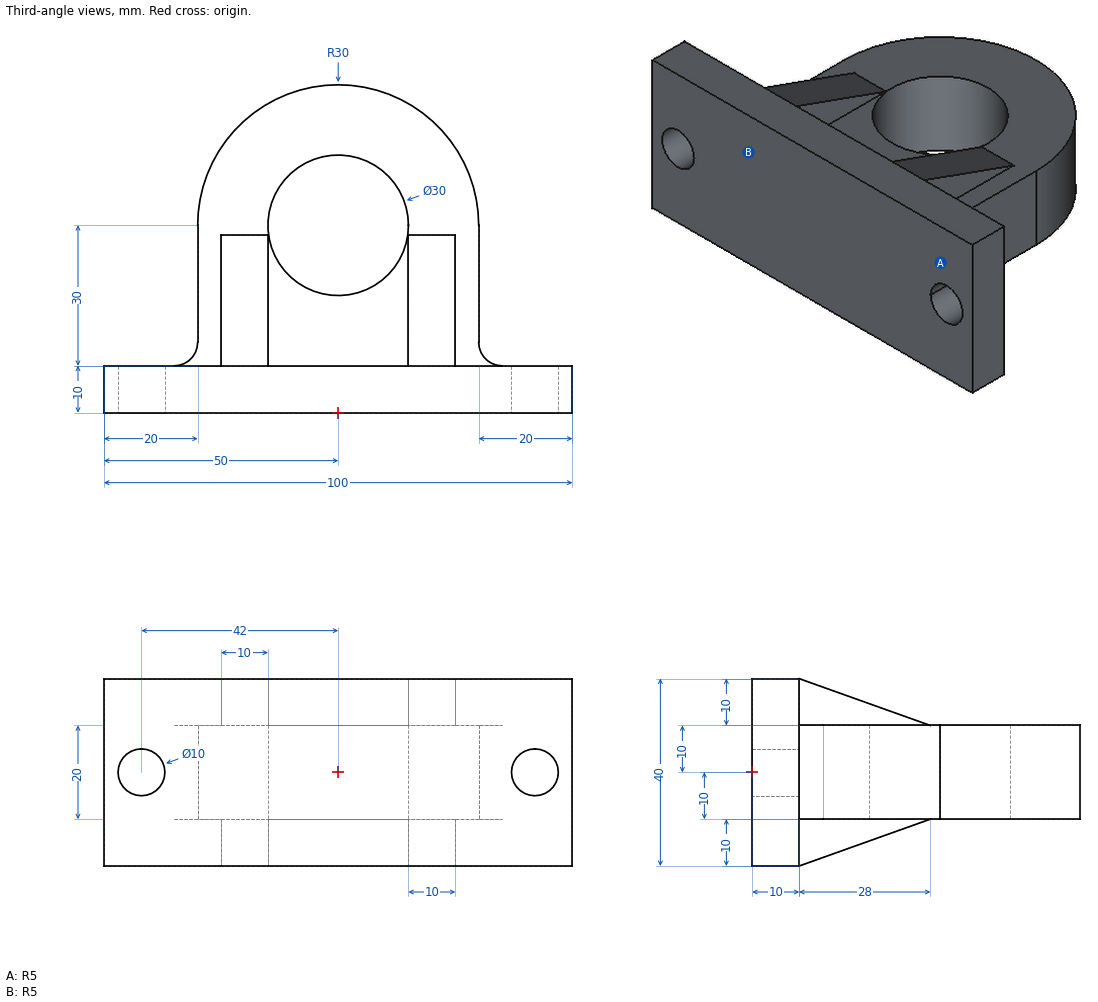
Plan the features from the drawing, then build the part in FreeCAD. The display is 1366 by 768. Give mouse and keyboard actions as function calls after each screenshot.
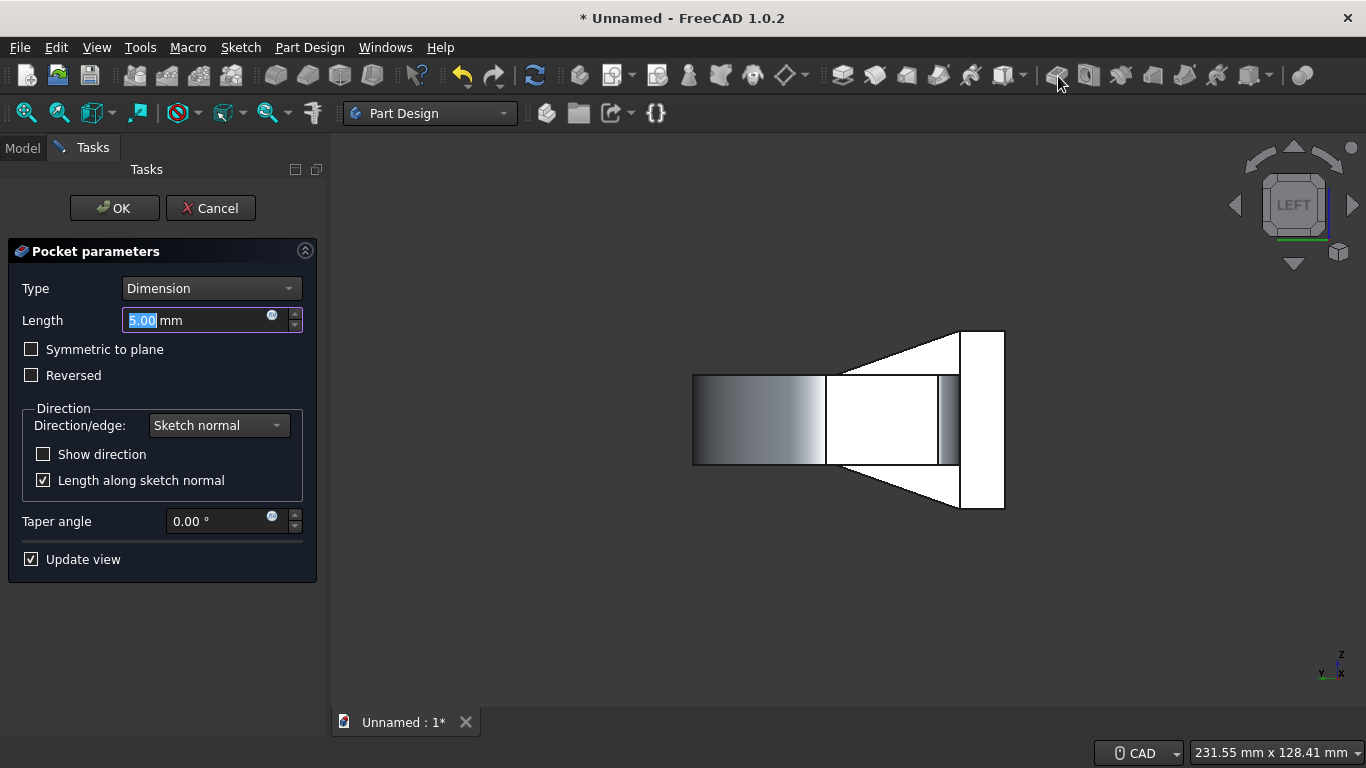
click(212, 288)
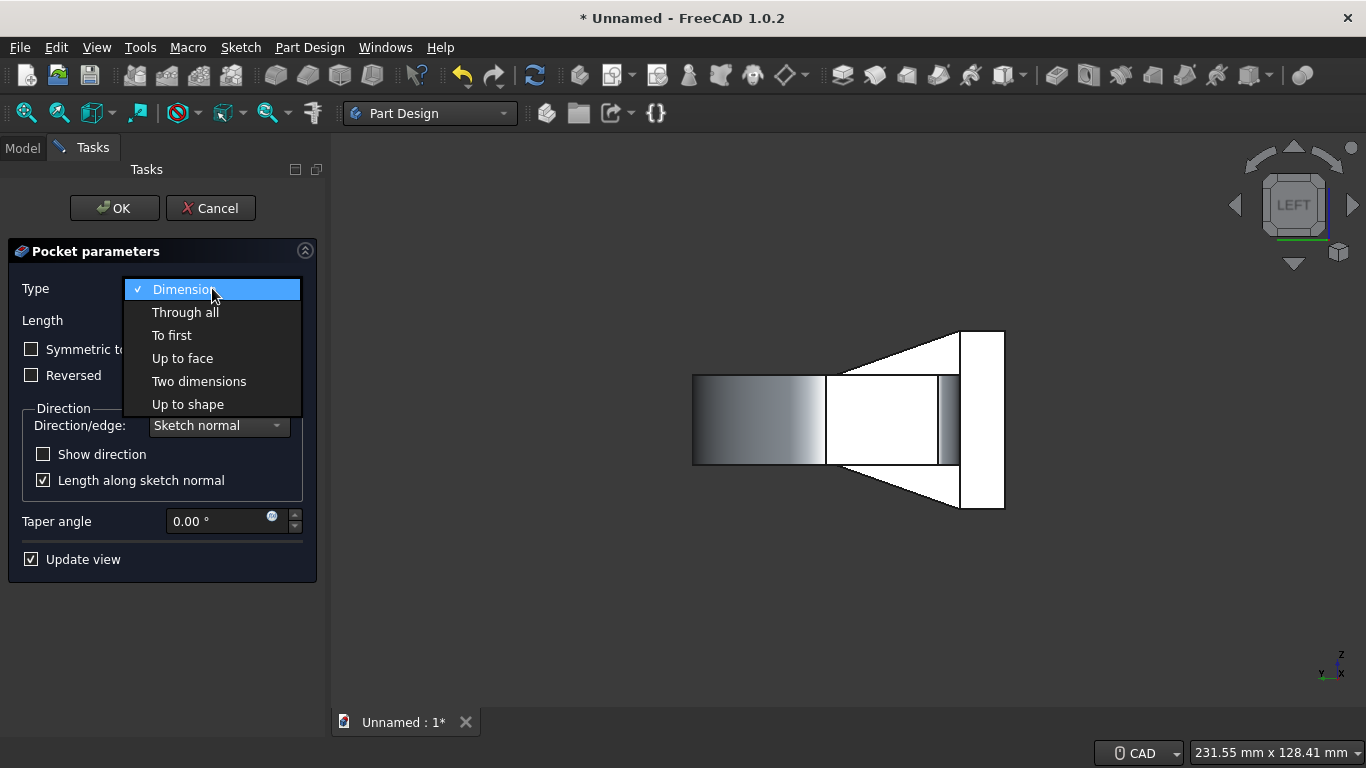
click(212, 312)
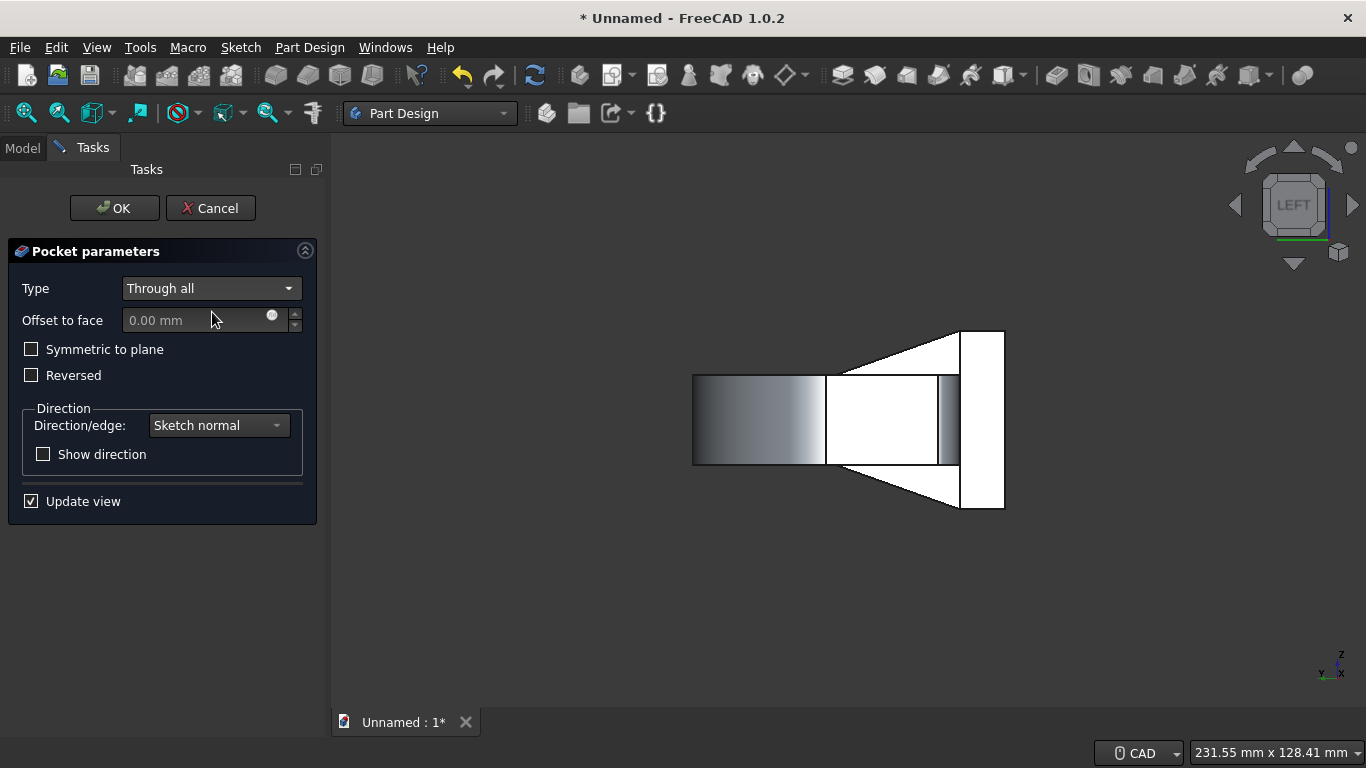
click(115, 208)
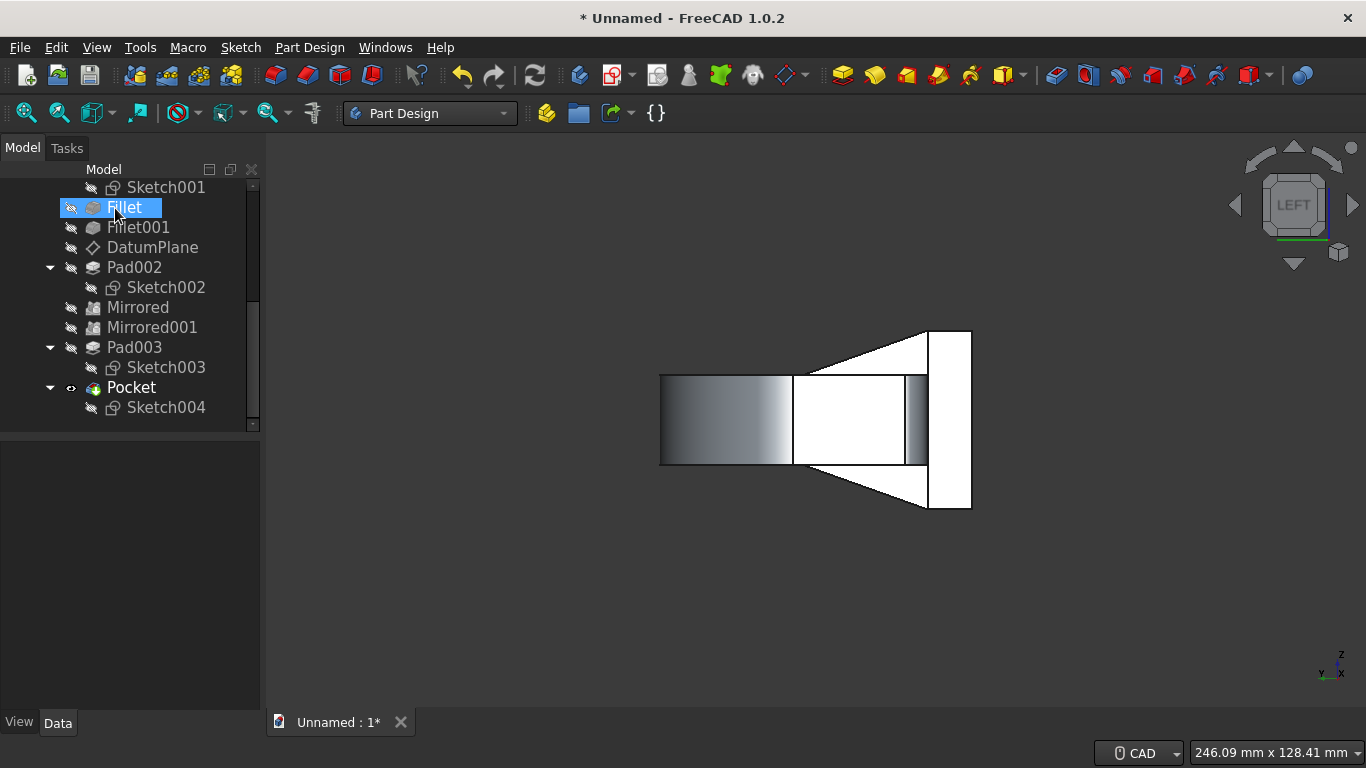
click(28, 114)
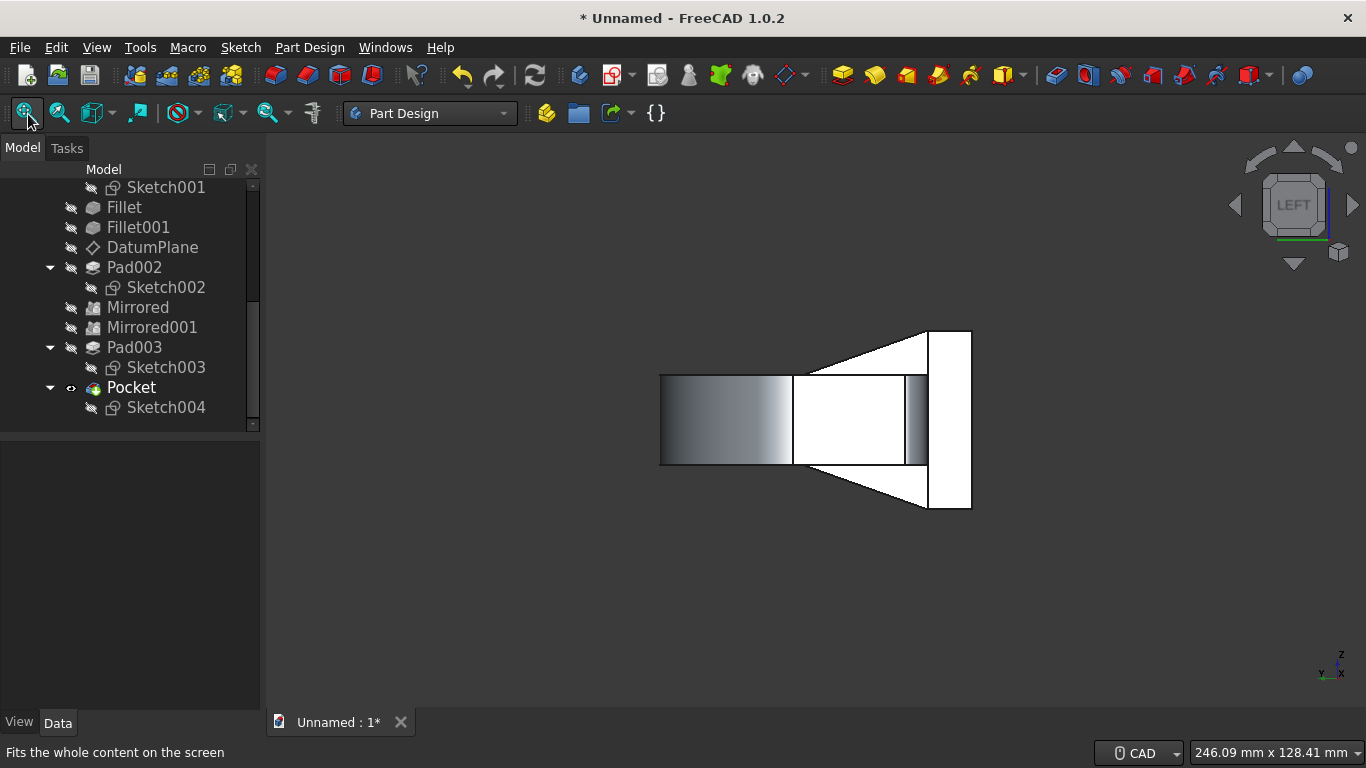
click(116, 388)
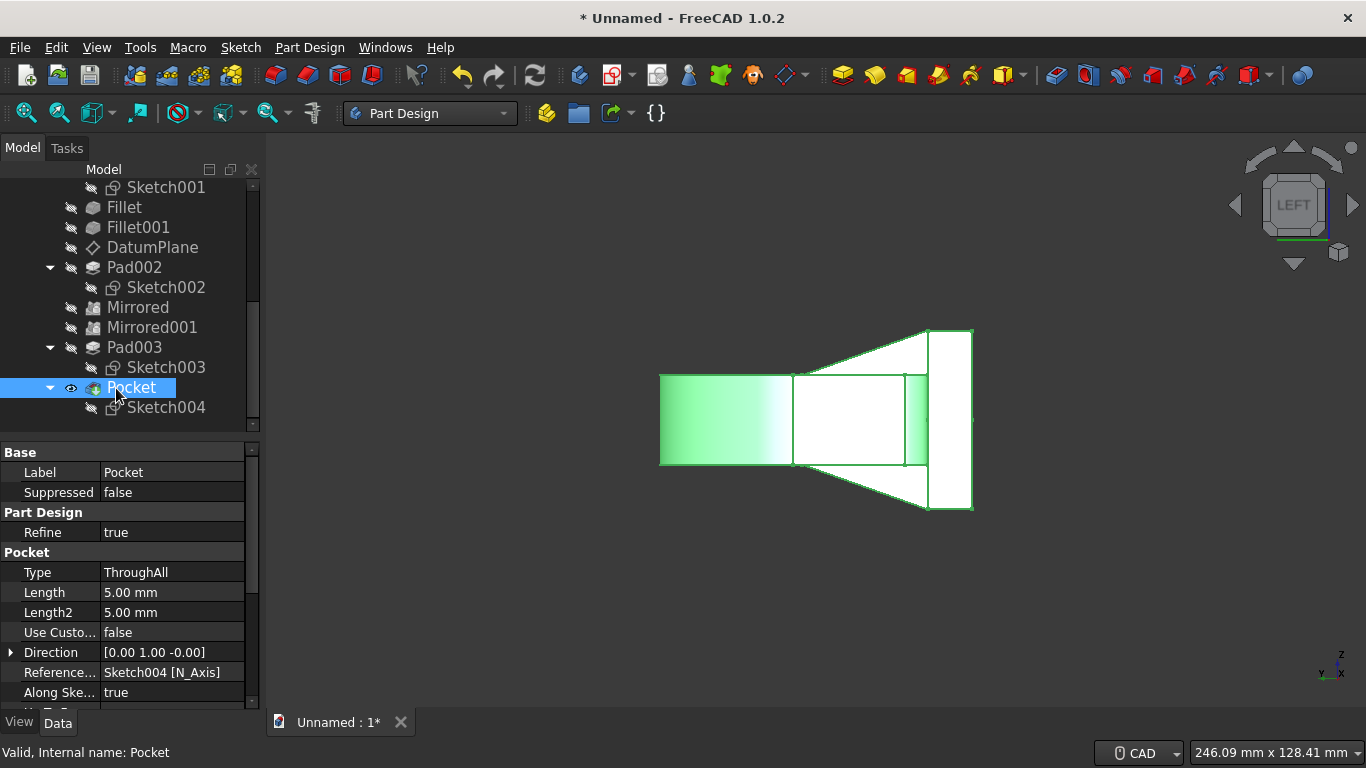
click(136, 76)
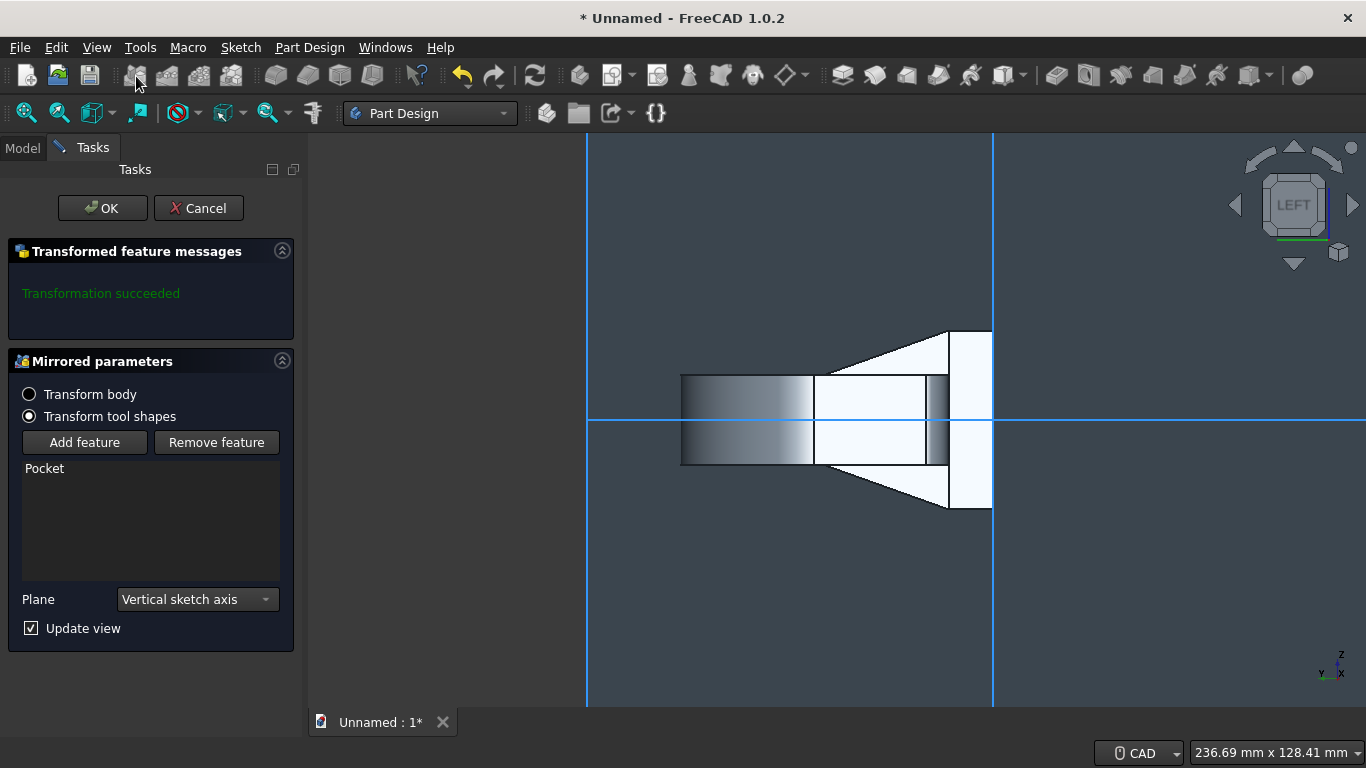
click(198, 600)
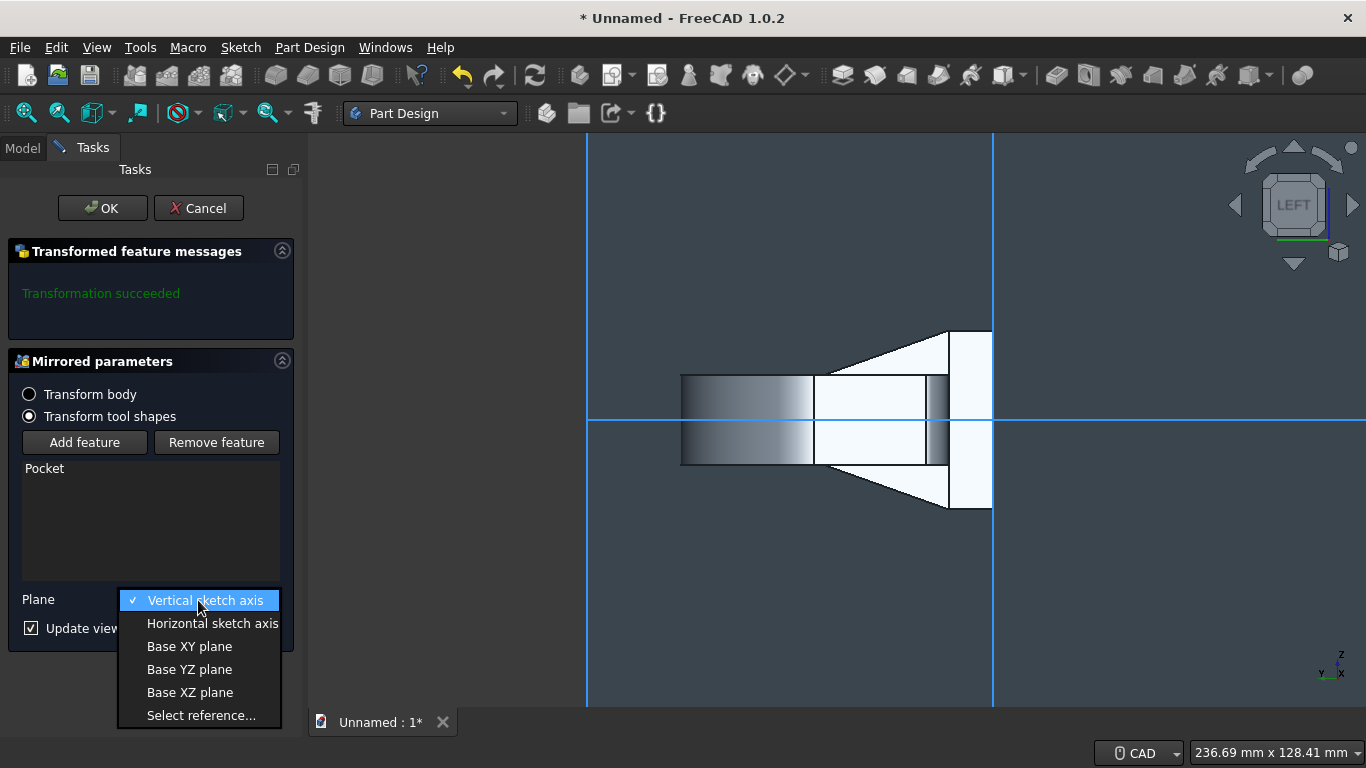
click(198, 670)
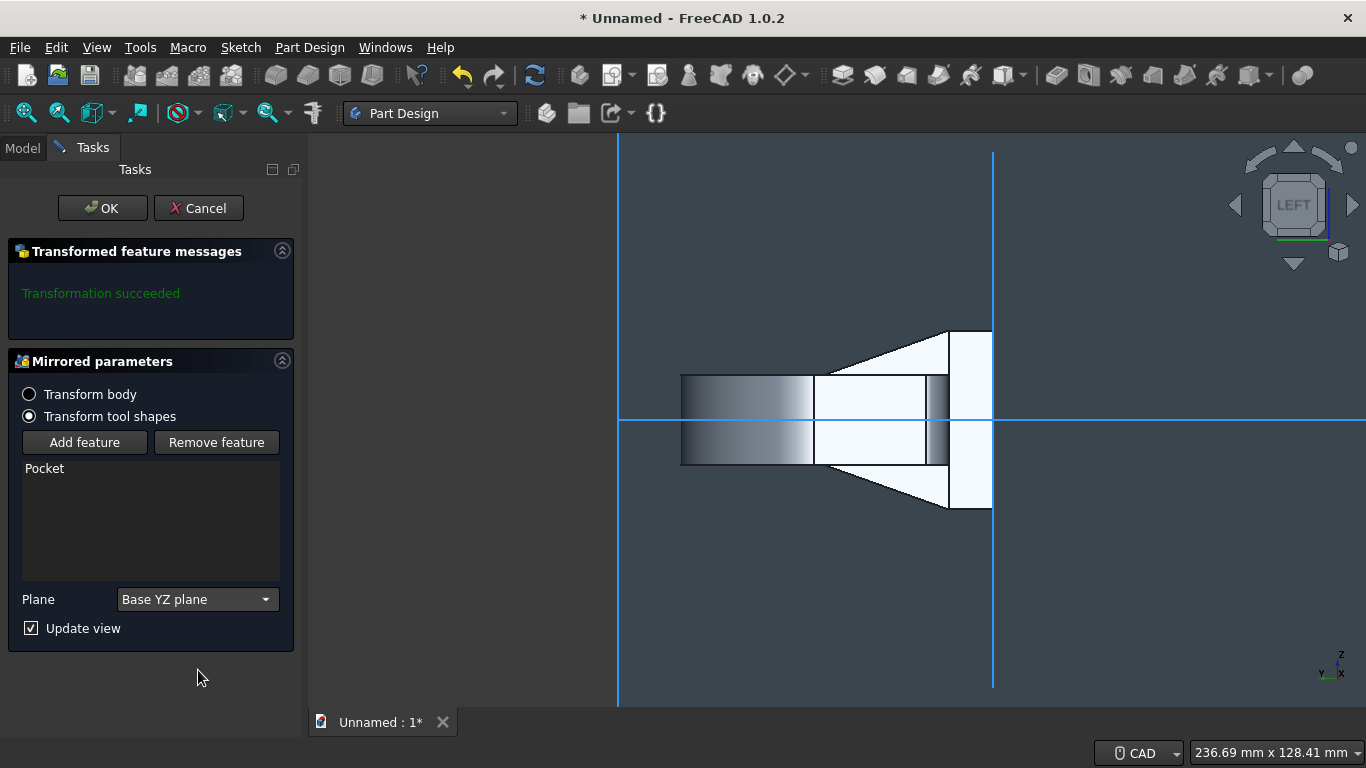
click(103, 208)